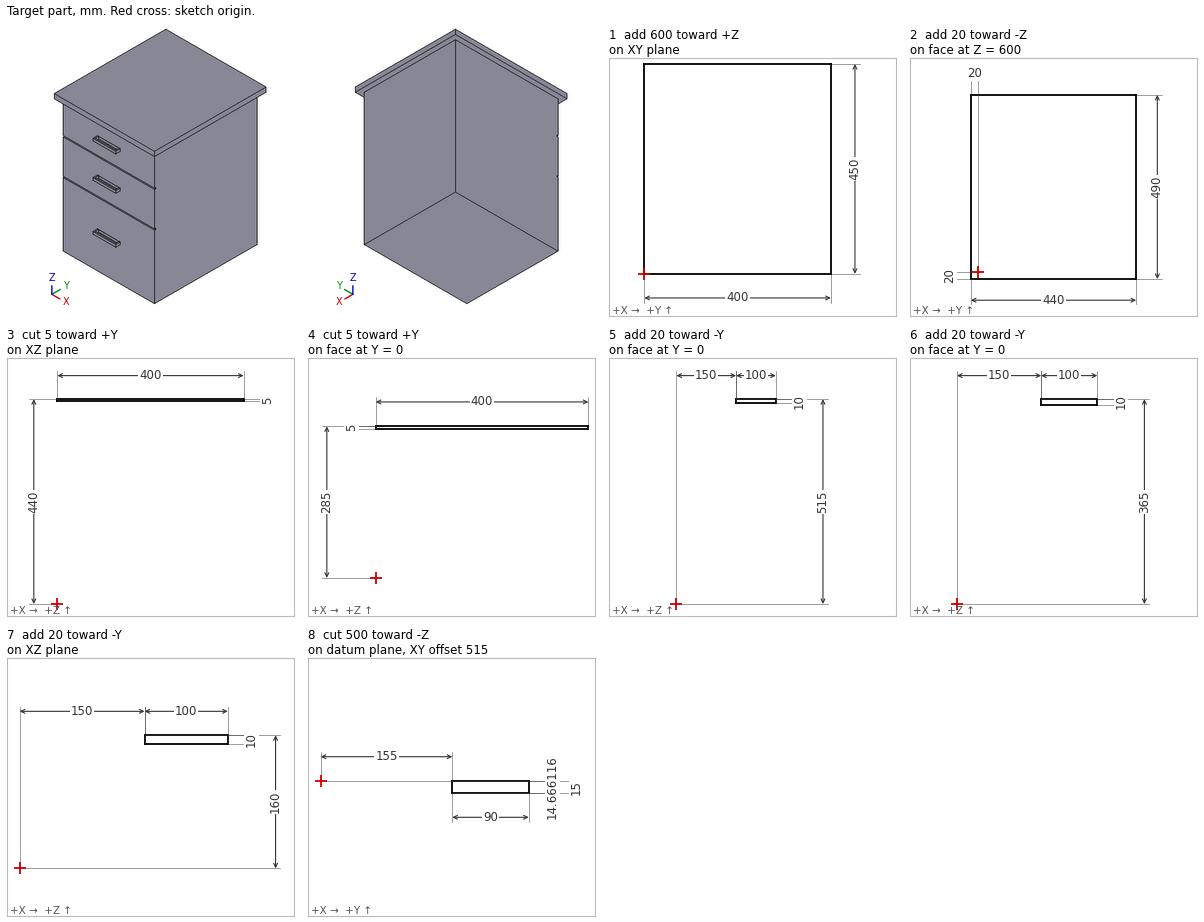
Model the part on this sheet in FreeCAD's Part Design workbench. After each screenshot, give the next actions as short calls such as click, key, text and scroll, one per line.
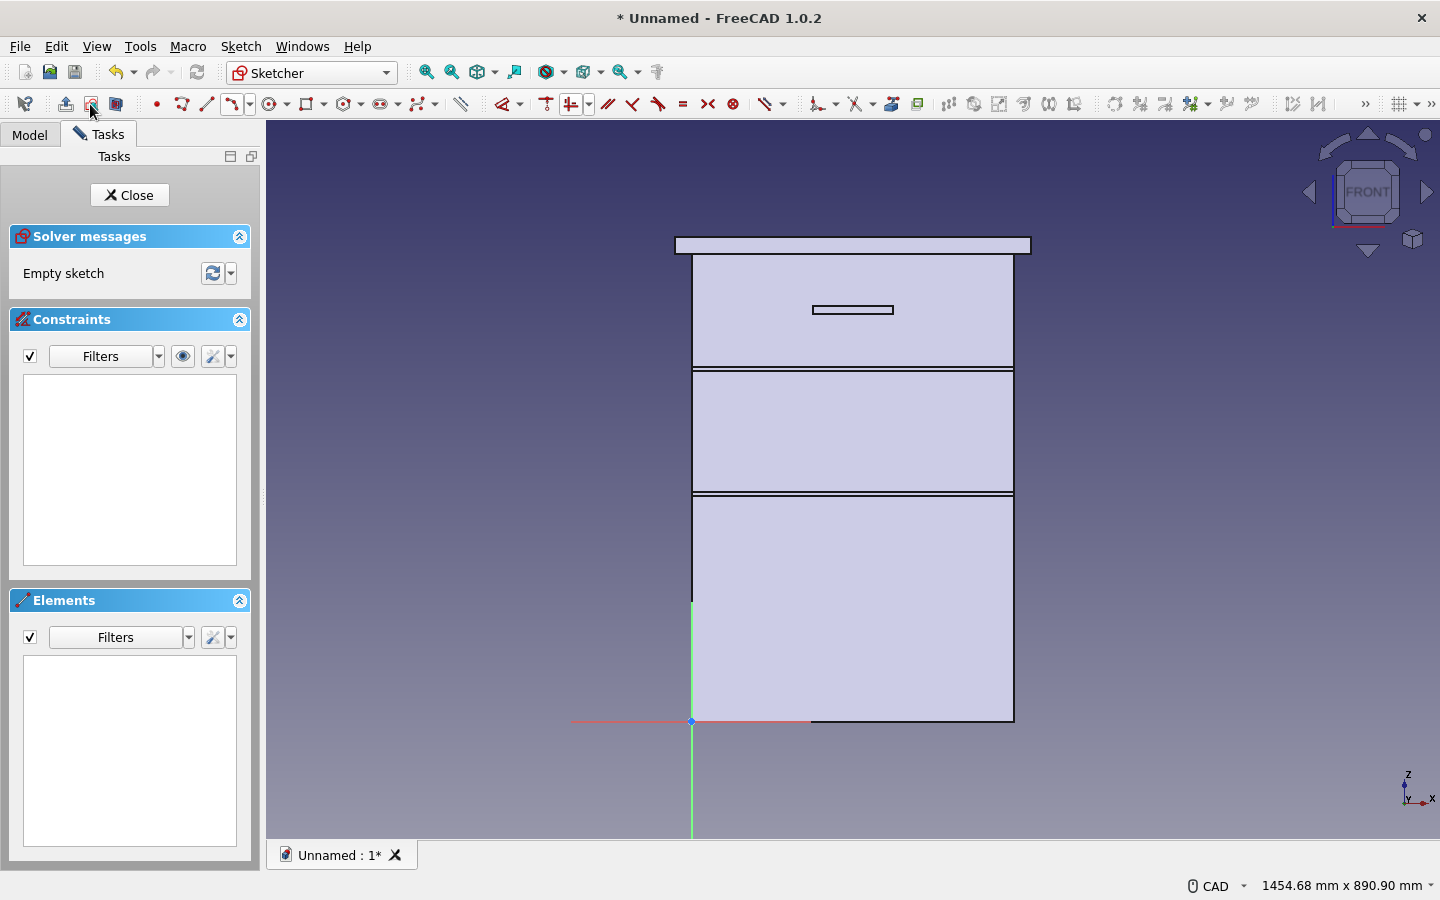
click(116, 104)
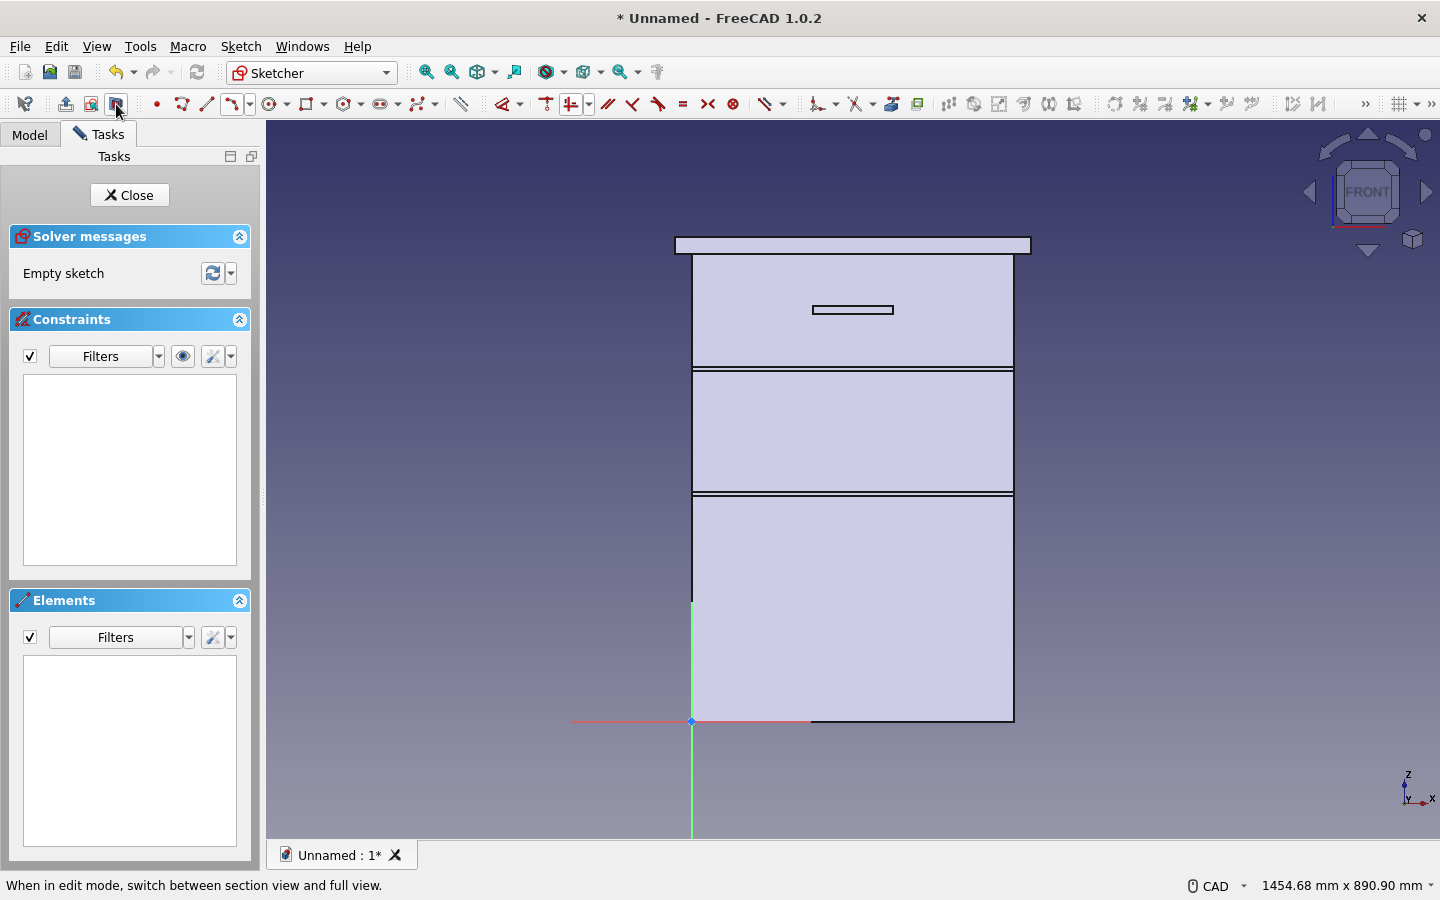
scroll(862, 425, up, 11)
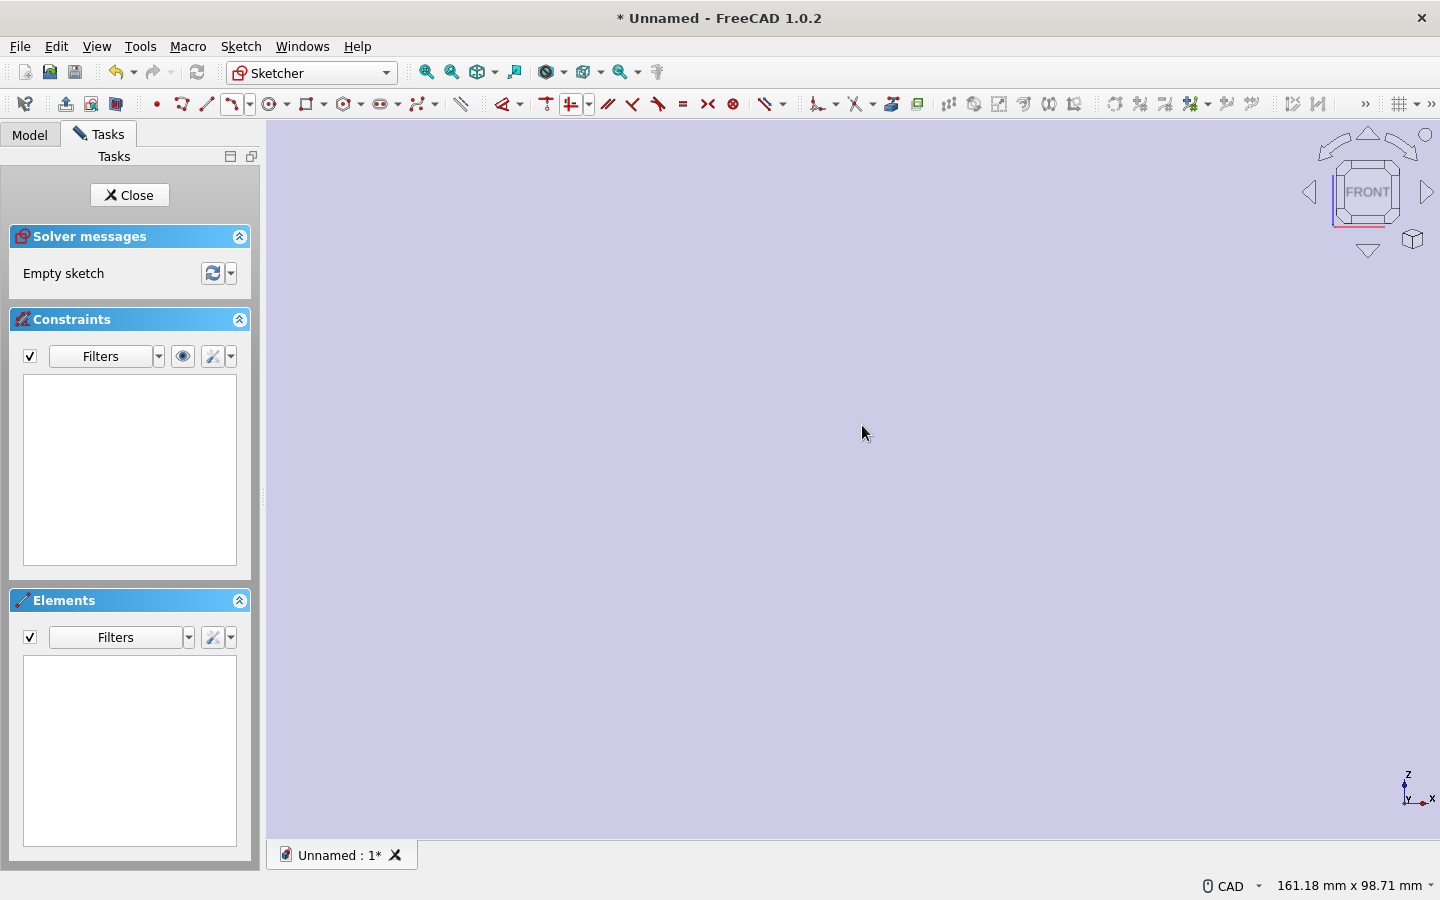
click(306, 104)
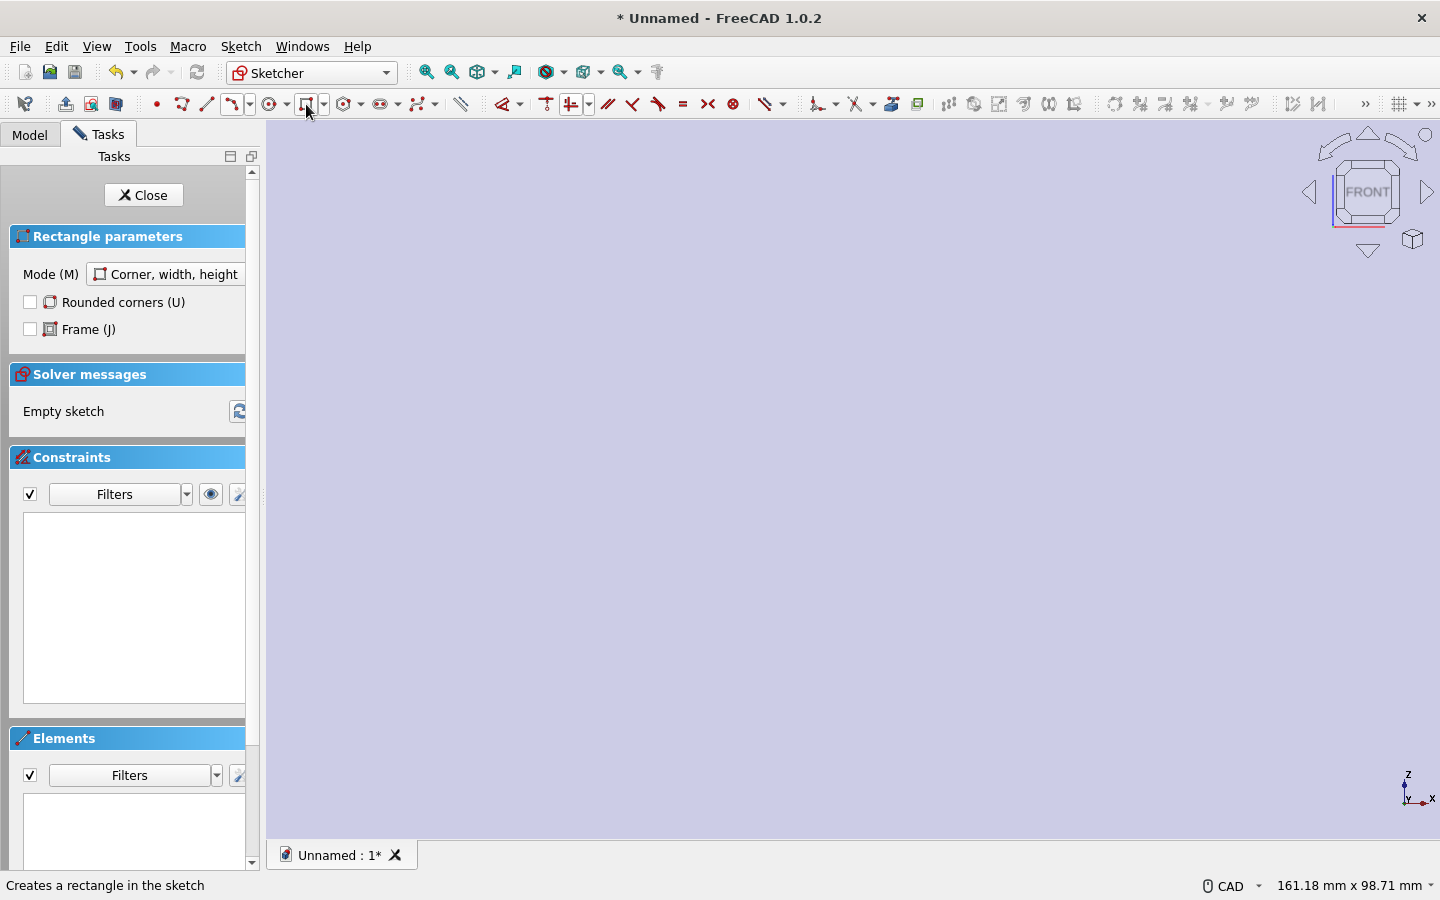
click(413, 440)
move(1141, 513)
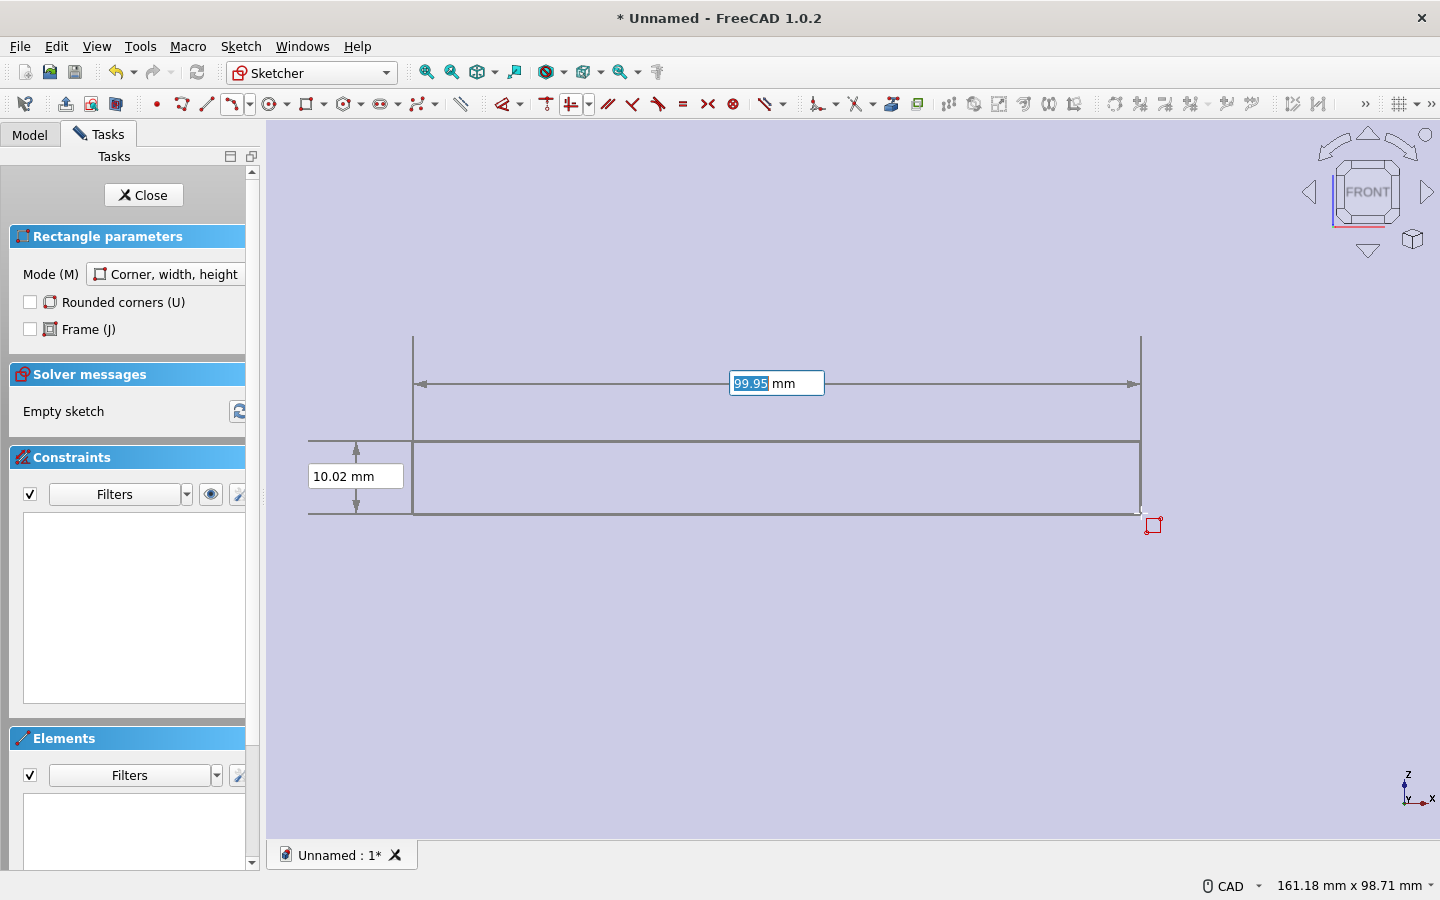
text(100)
key(Tab)
text(10)
key(Return)
key(Escape)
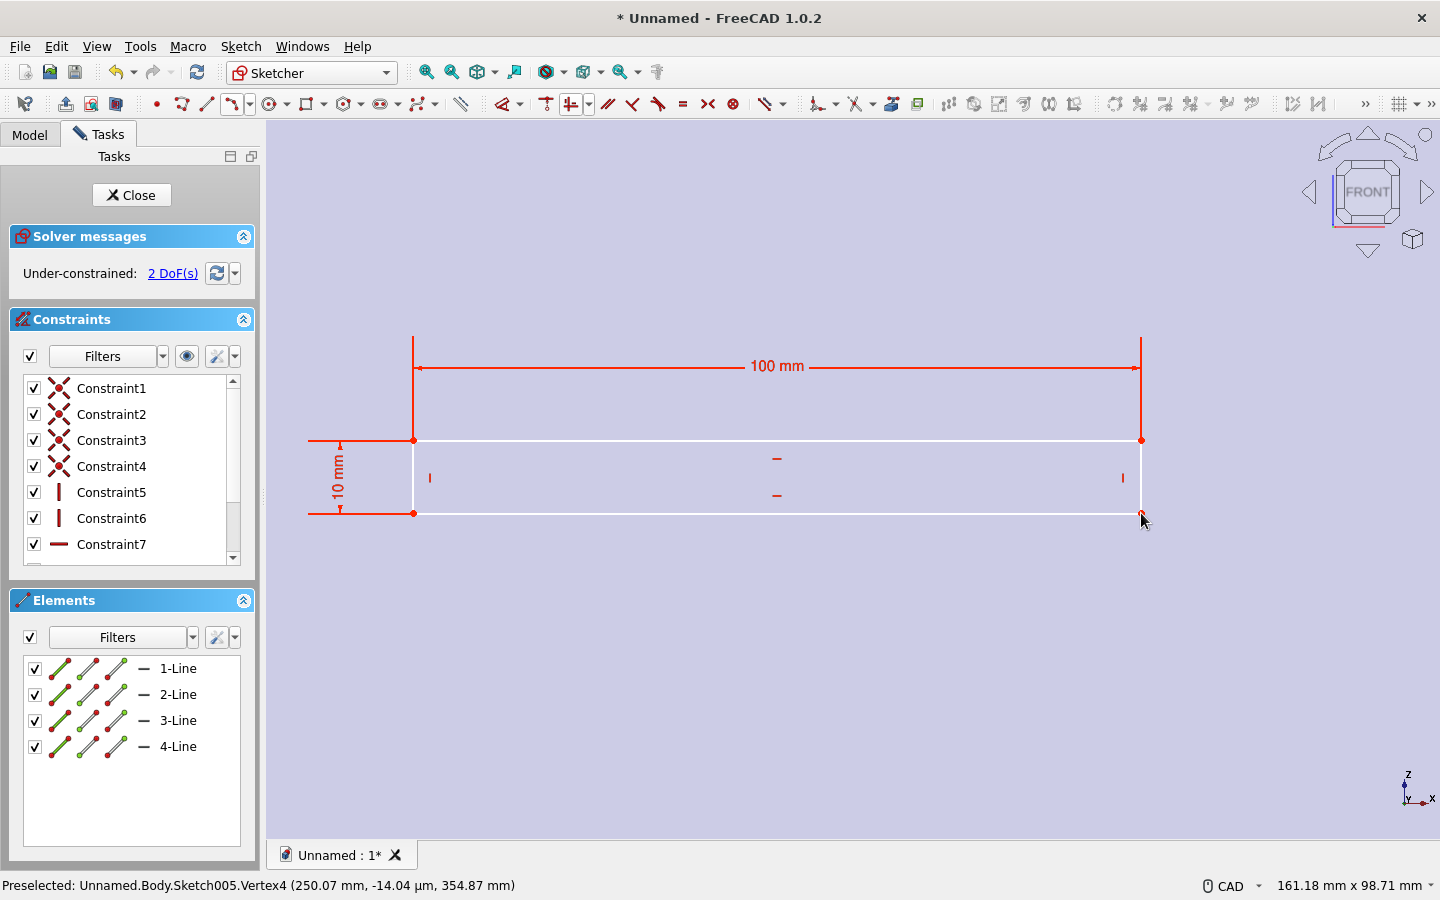
click(502, 104)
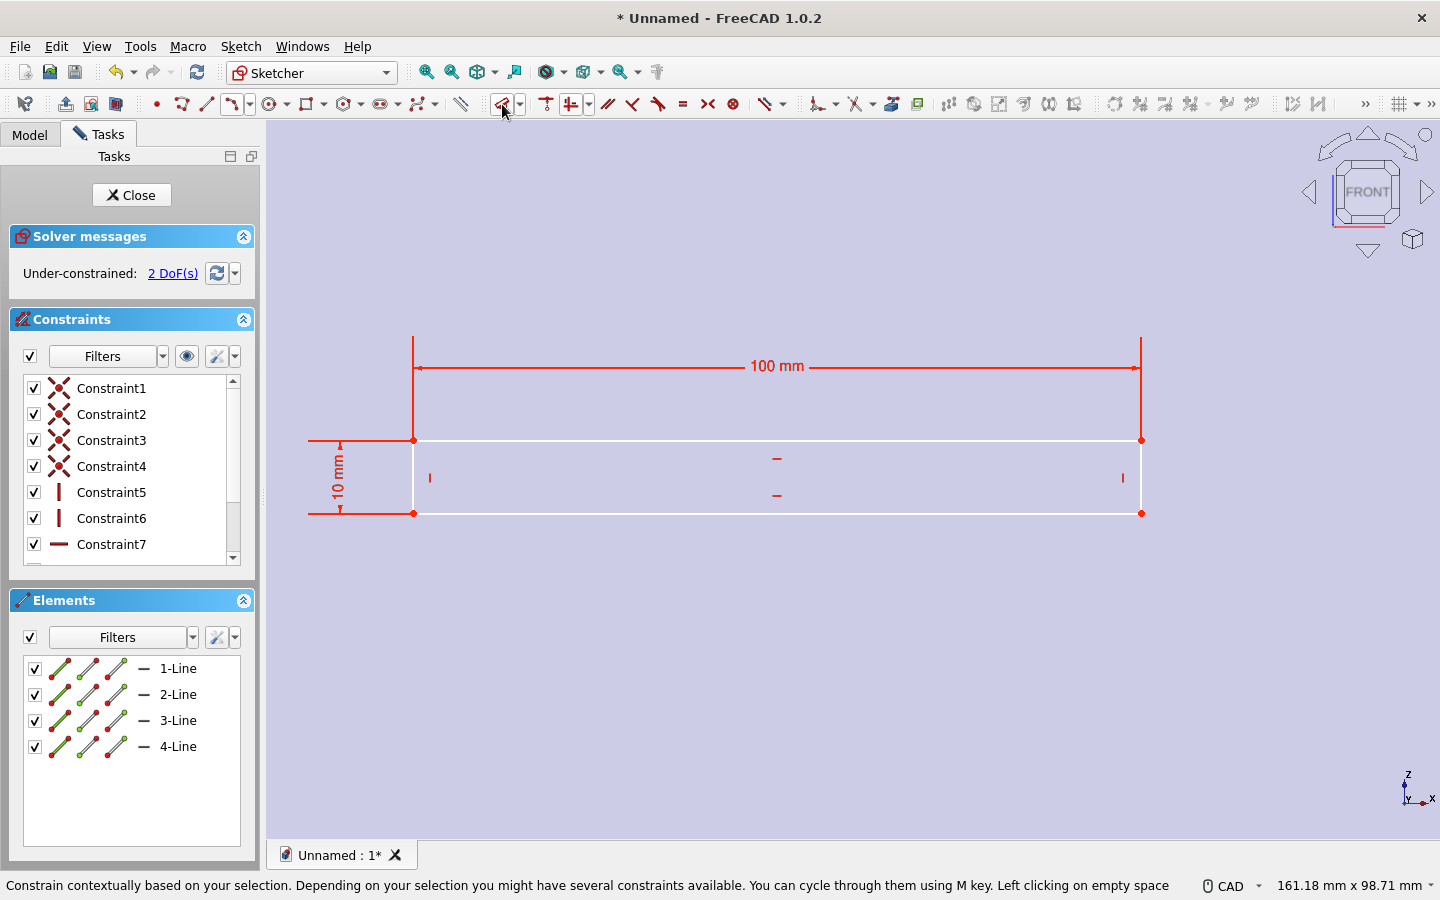
click(413, 441)
click(354, 407)